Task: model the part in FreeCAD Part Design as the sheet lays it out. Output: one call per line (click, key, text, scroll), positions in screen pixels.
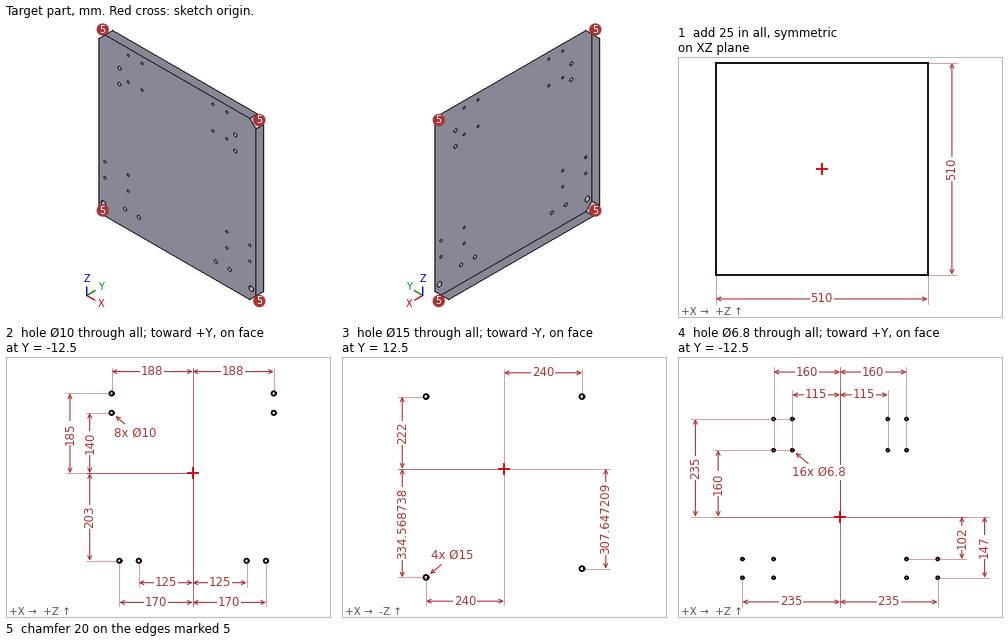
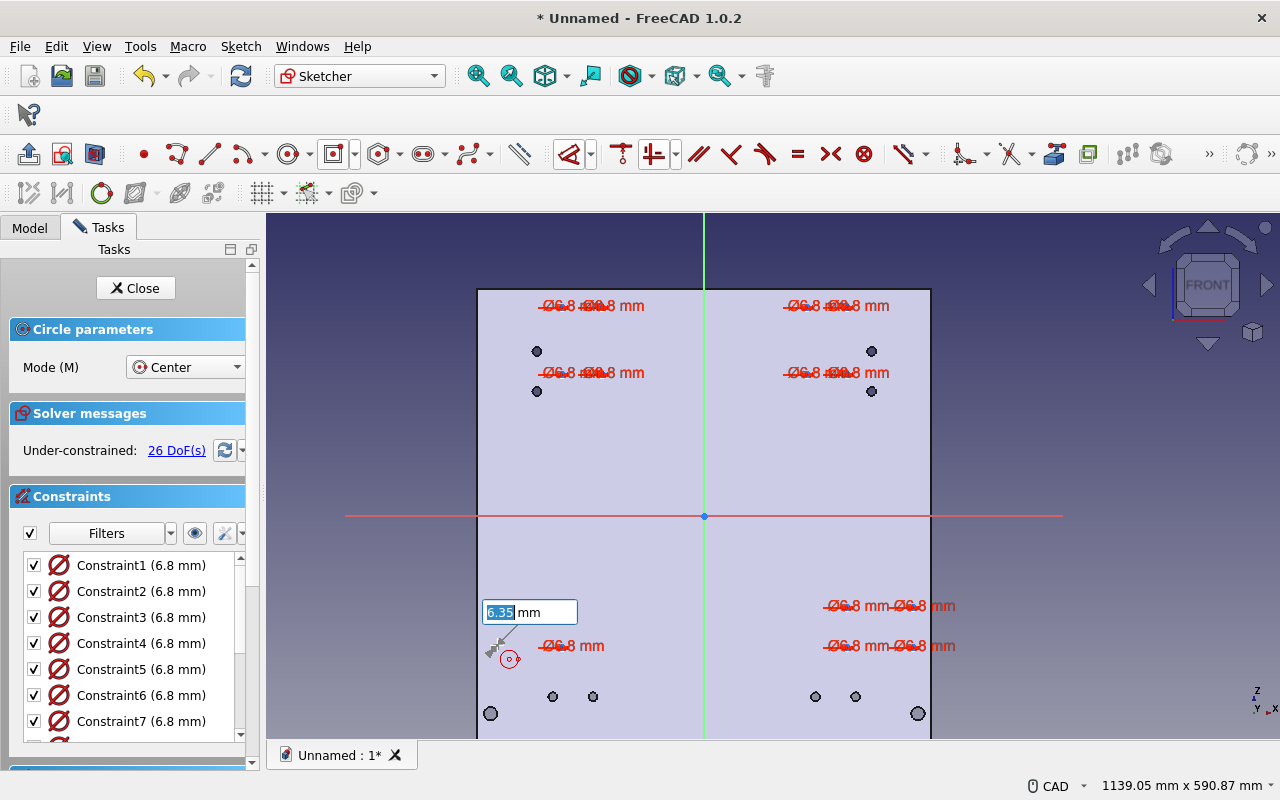
text(6.8)
key(Return)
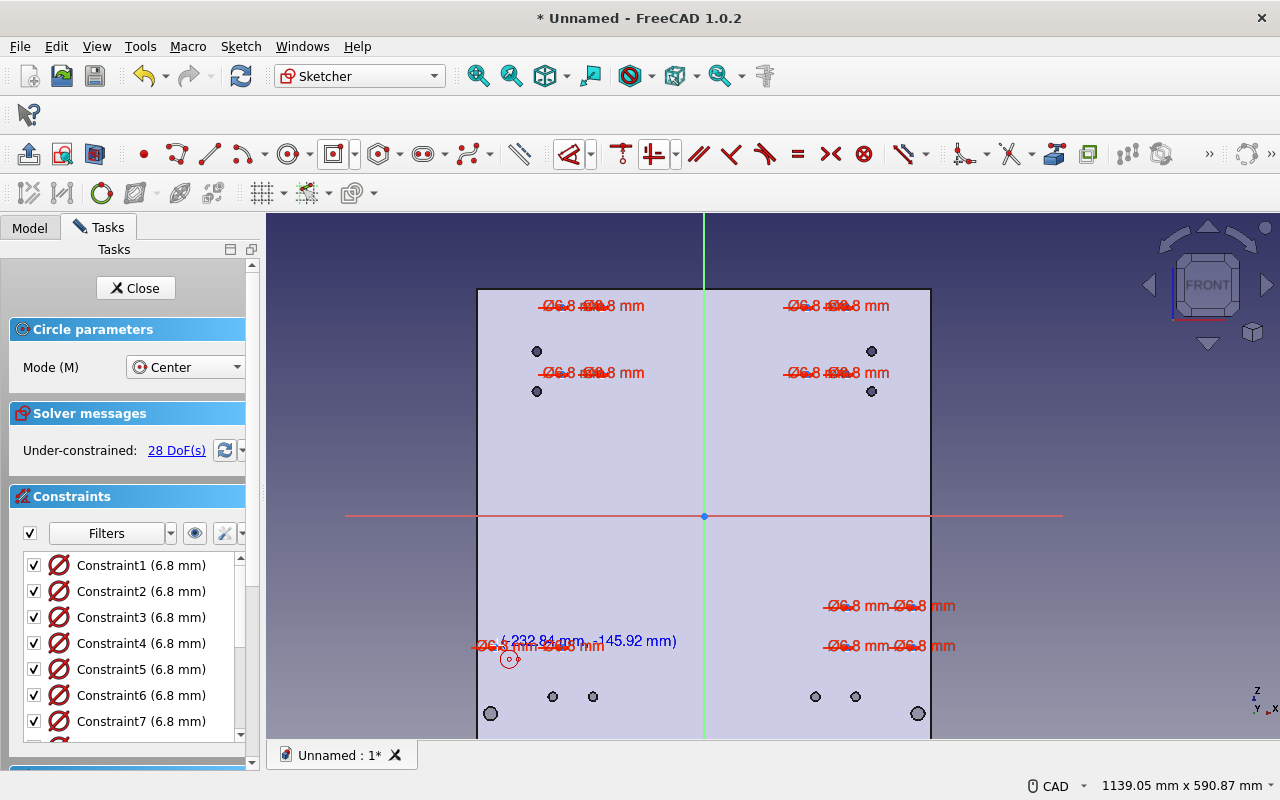
scroll(495, 607, up, 11)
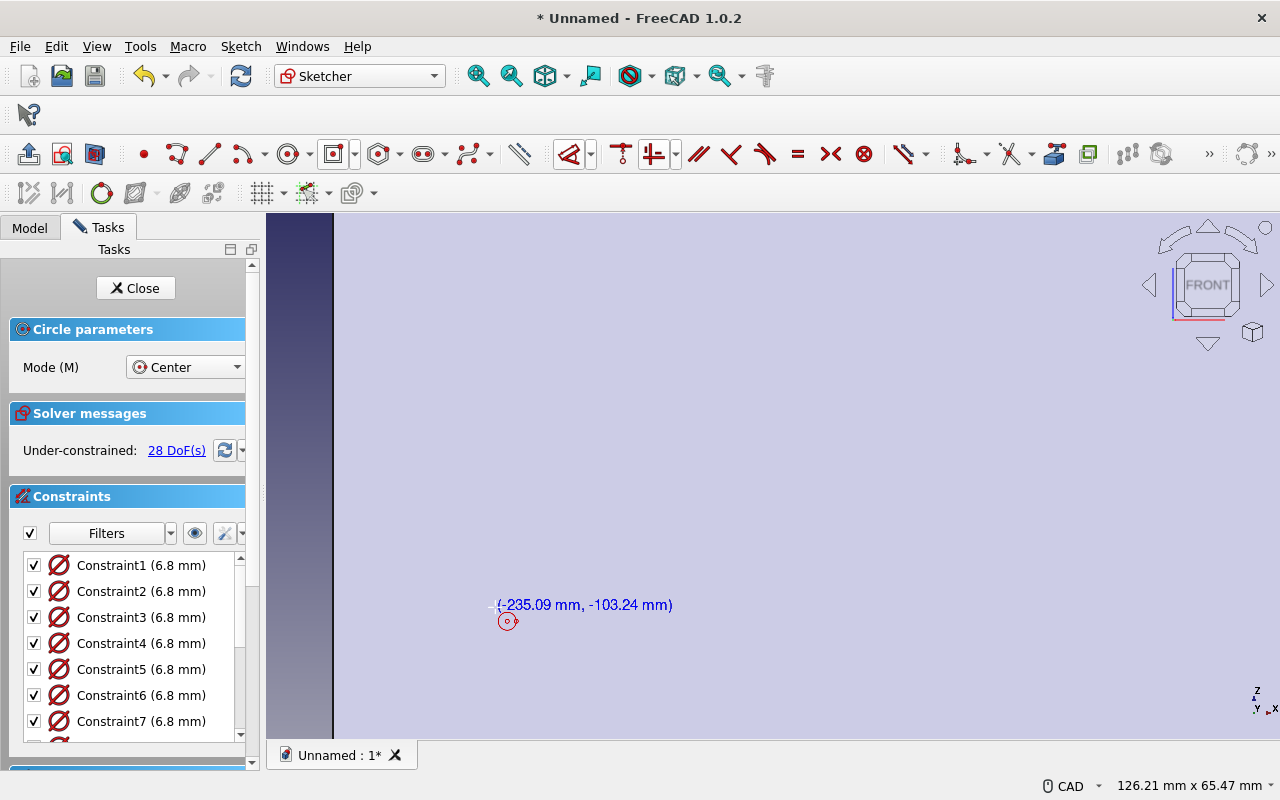
scroll(495, 607, down, 11)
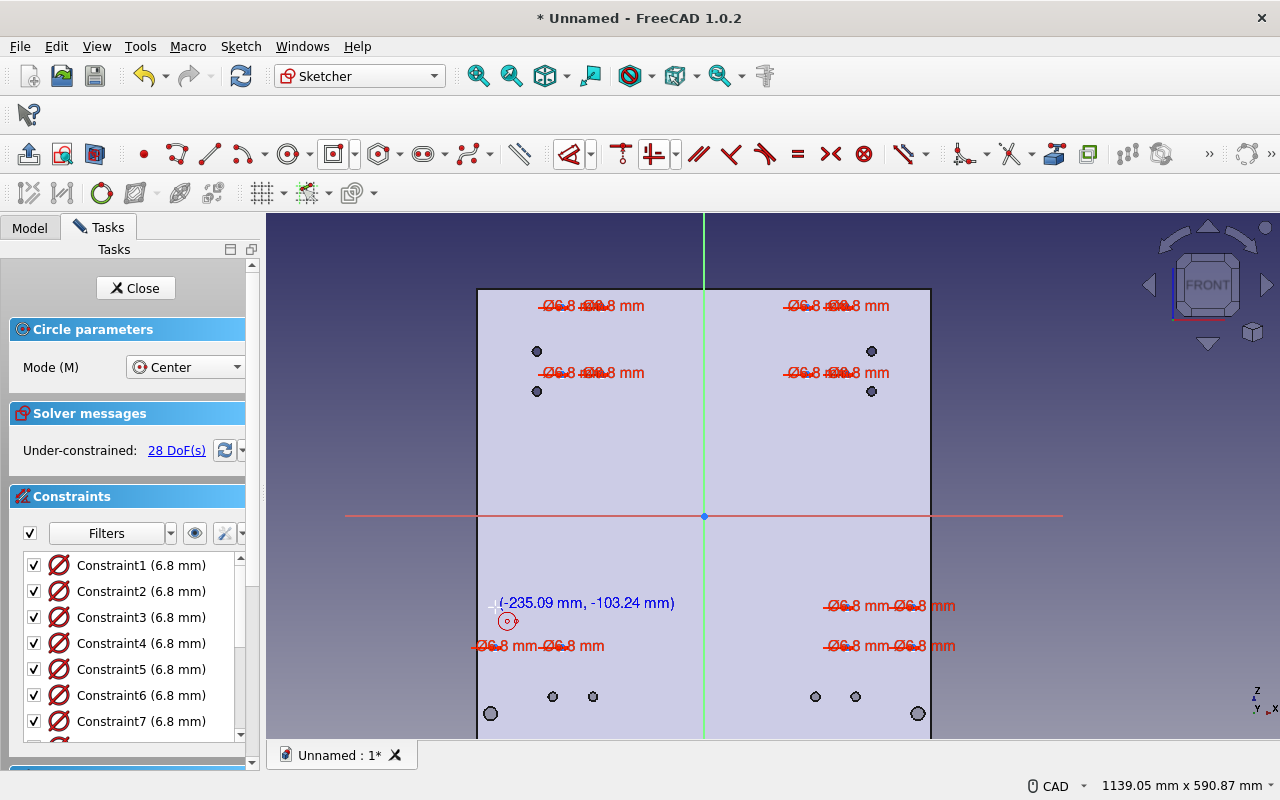
click(495, 607)
move(497, 605)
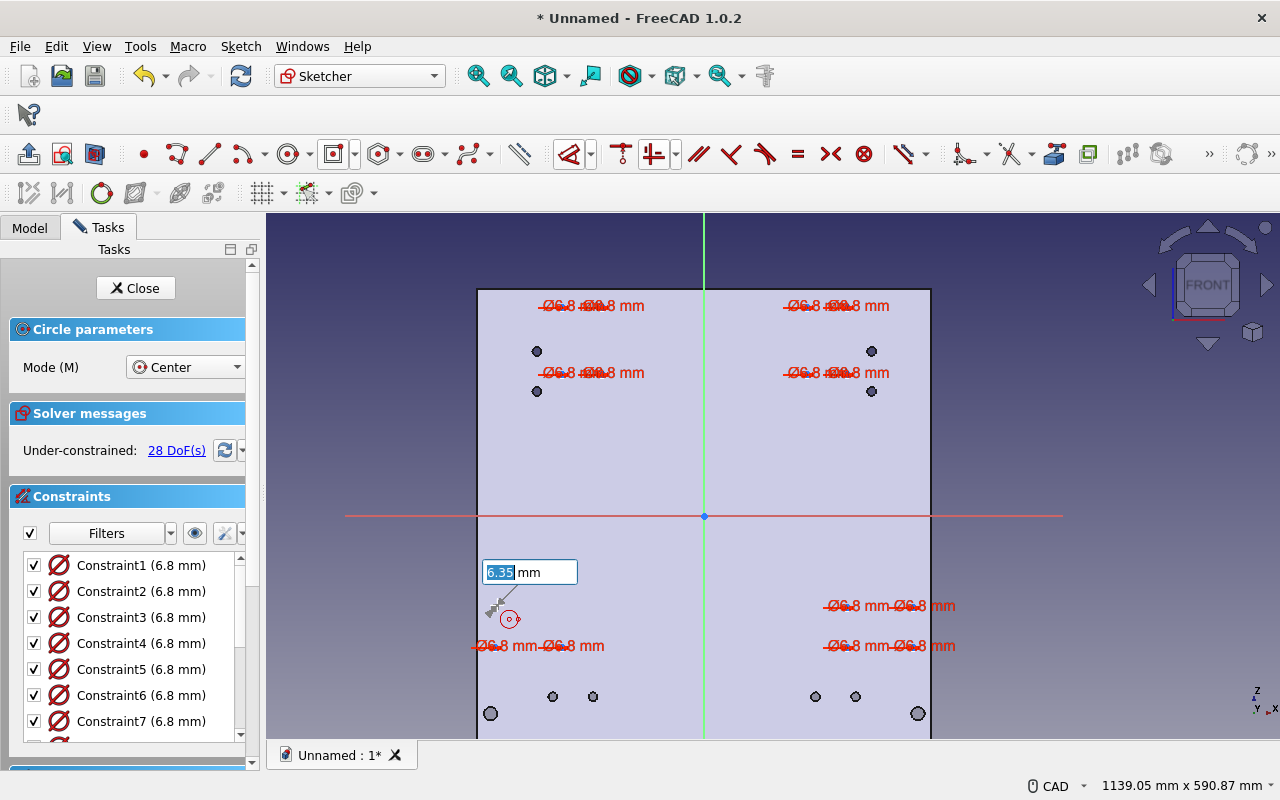
text(6.8)
key(Return)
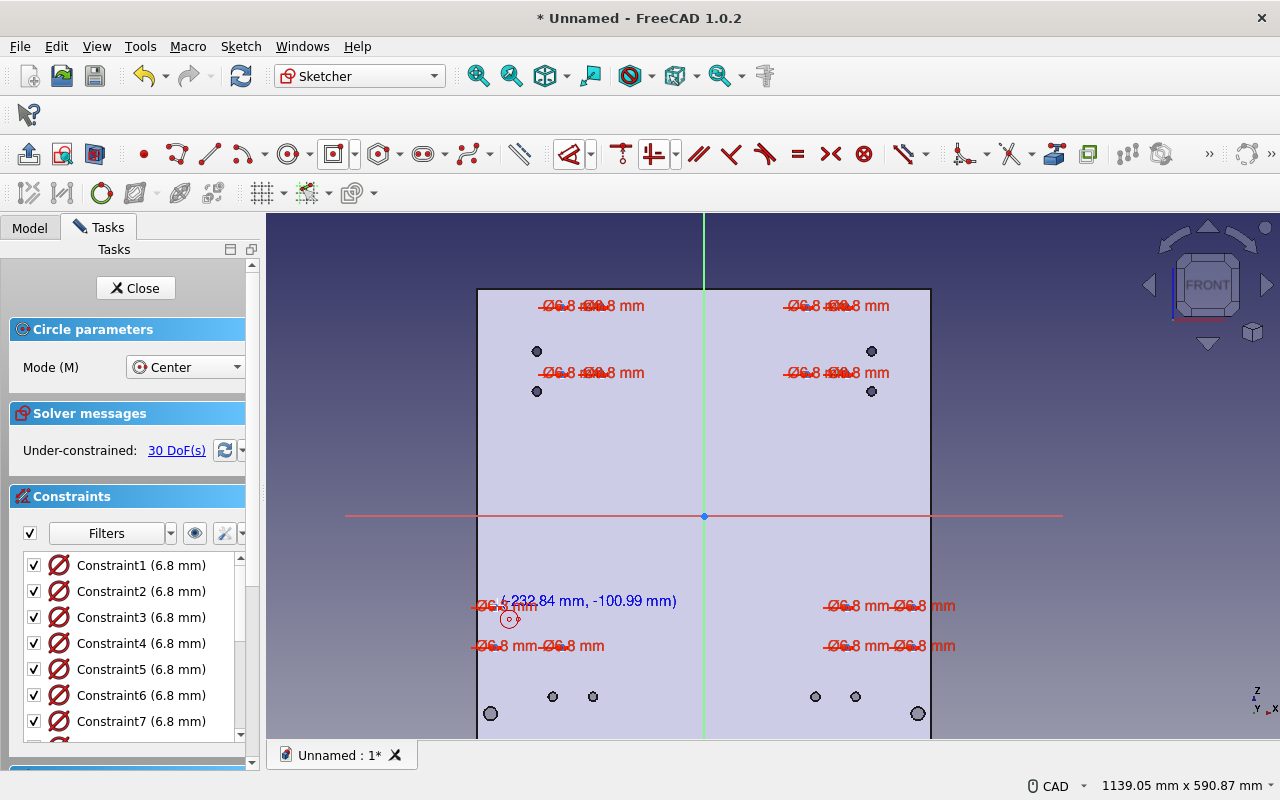
scroll(562, 607, up, 11)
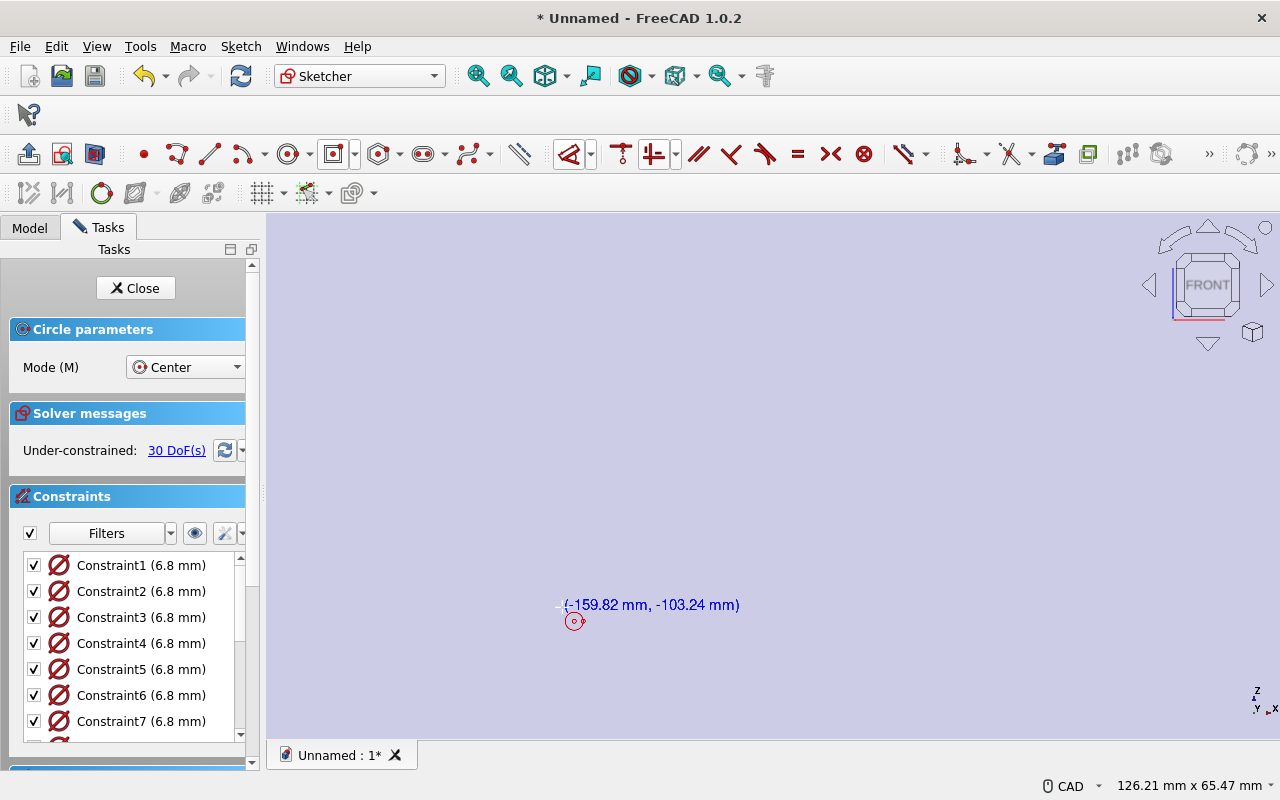
scroll(563, 607, down, 11)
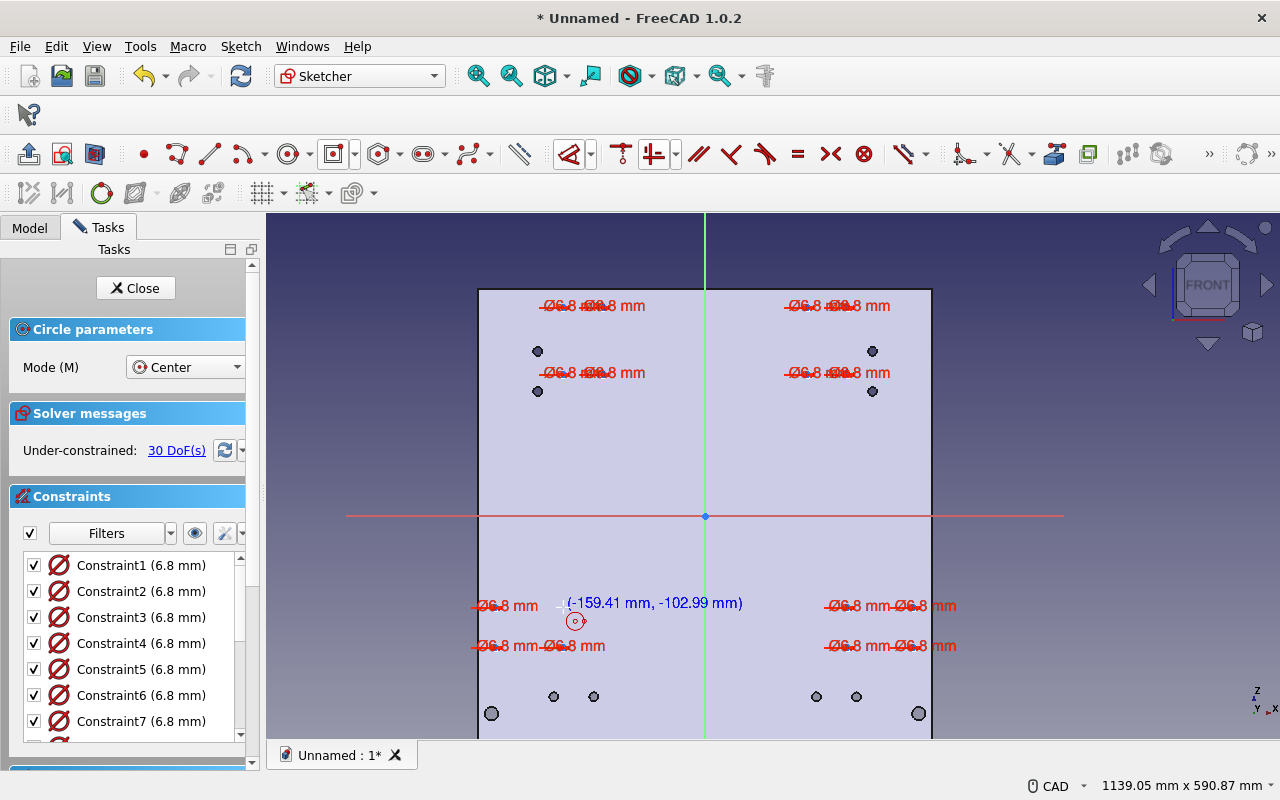
click(563, 607)
move(565, 605)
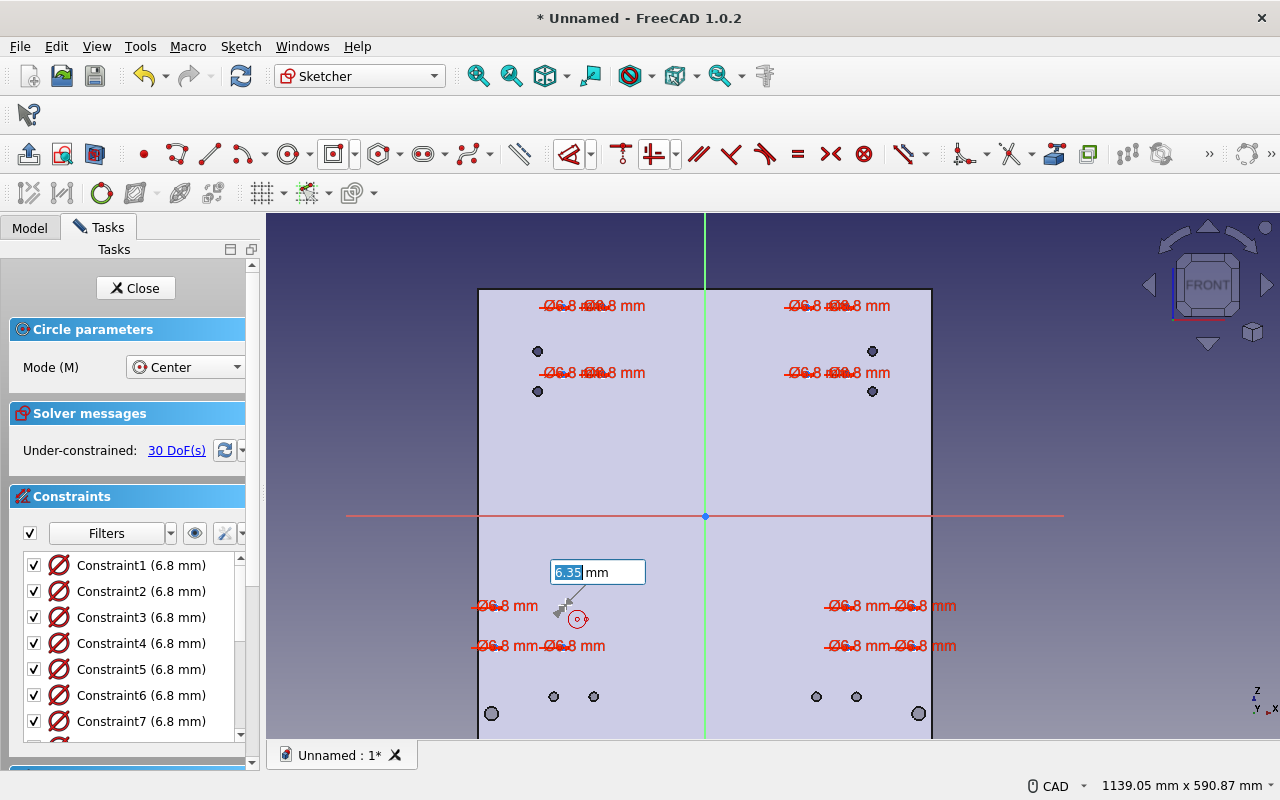
text(6.8)
key(Return)
key(Escape)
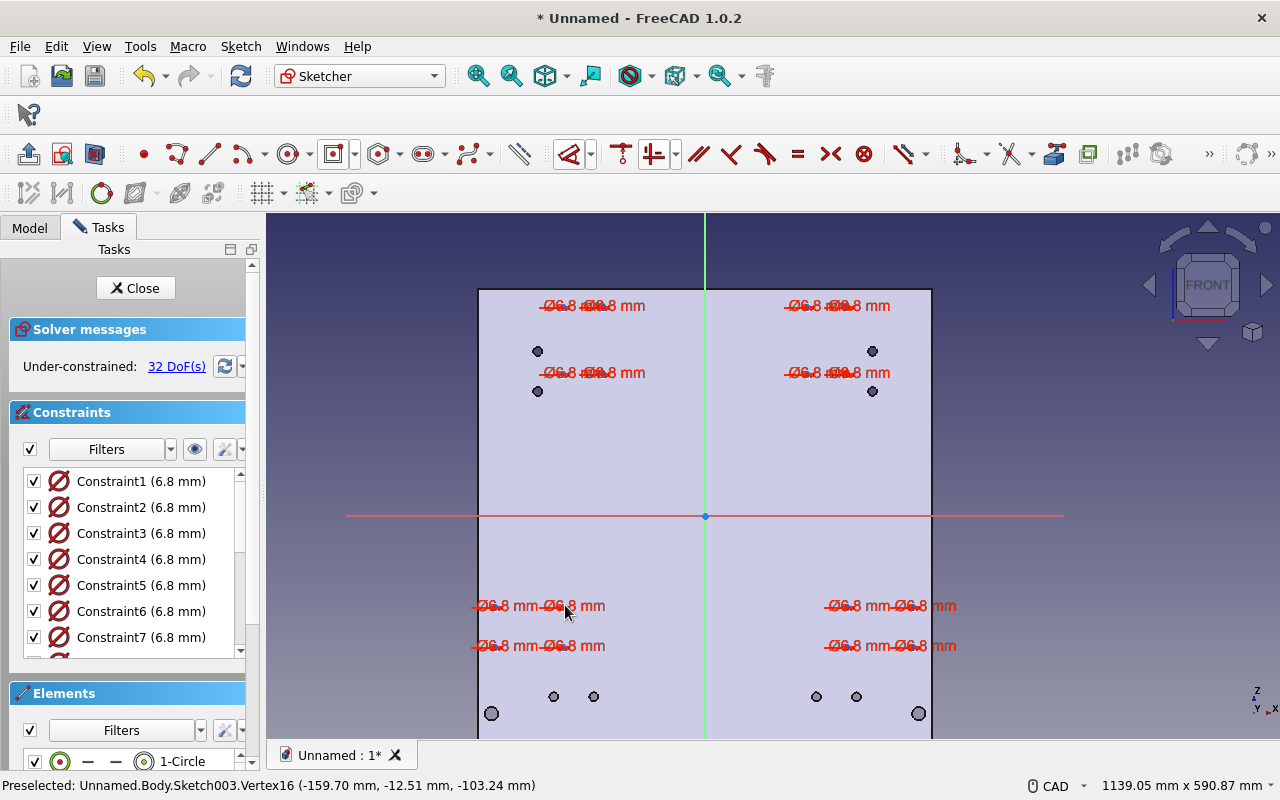
click(603, 375)